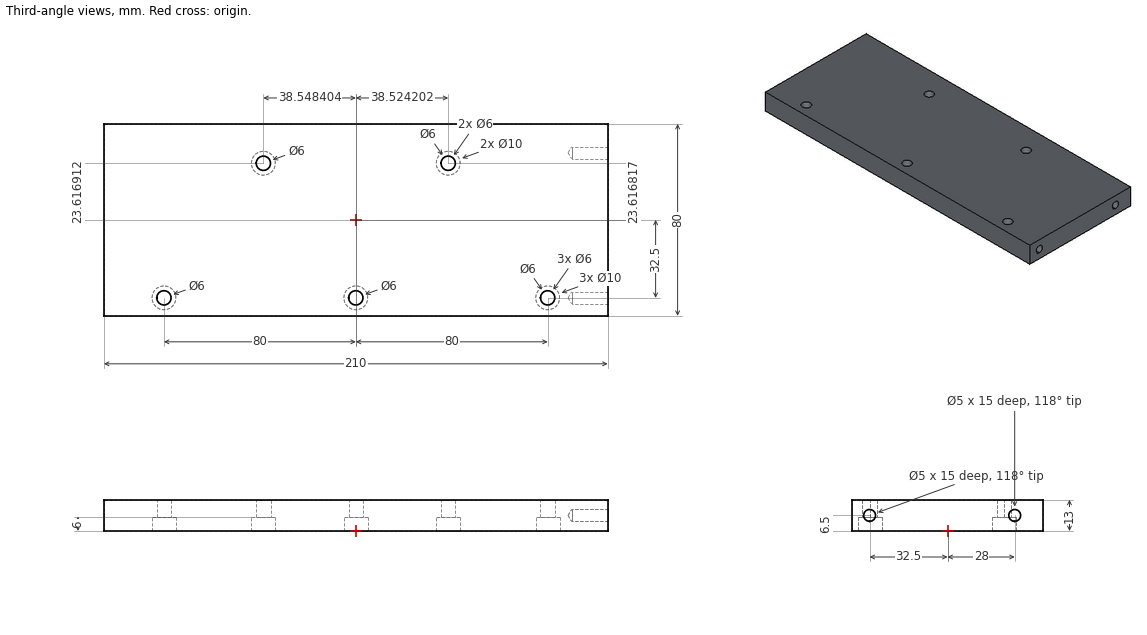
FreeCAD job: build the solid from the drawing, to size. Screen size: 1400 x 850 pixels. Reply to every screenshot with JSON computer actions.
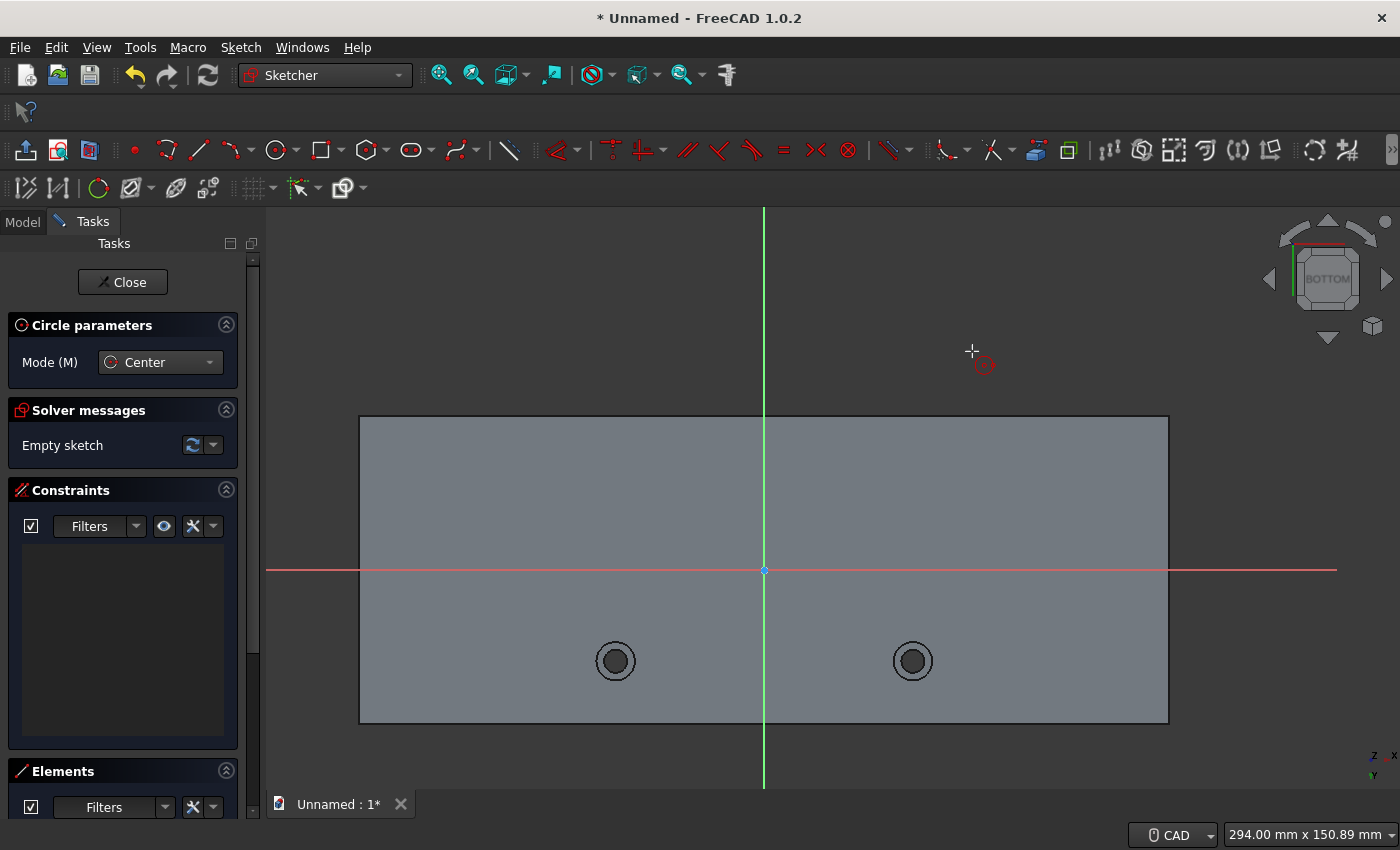
{"action": "left_click", "coordinate": [1073, 445]}
{"action": "left_click", "coordinate": [1087, 431]}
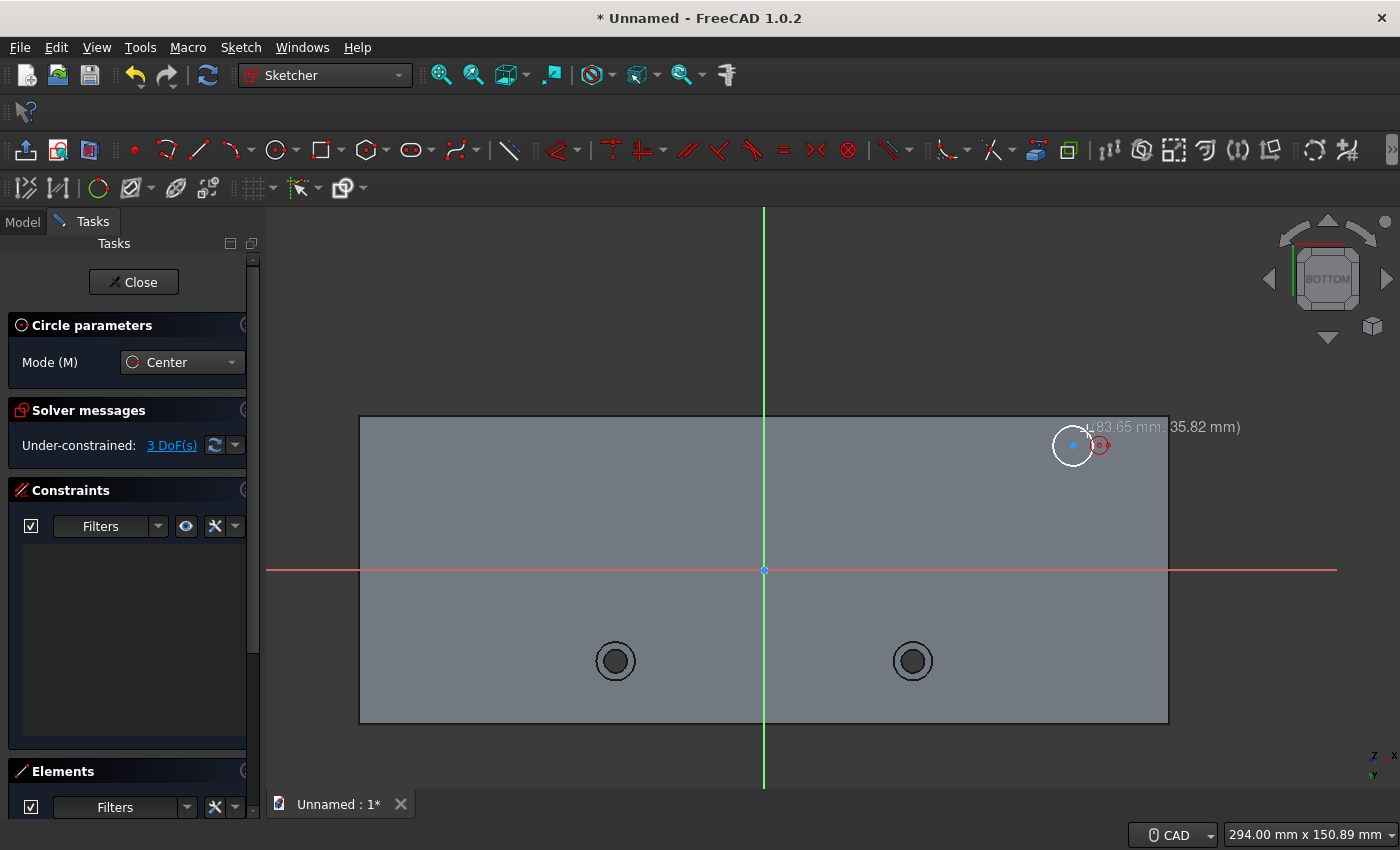
{"action": "left_click", "coordinate": [456, 445]}
{"action": "left_click", "coordinate": [469, 431]}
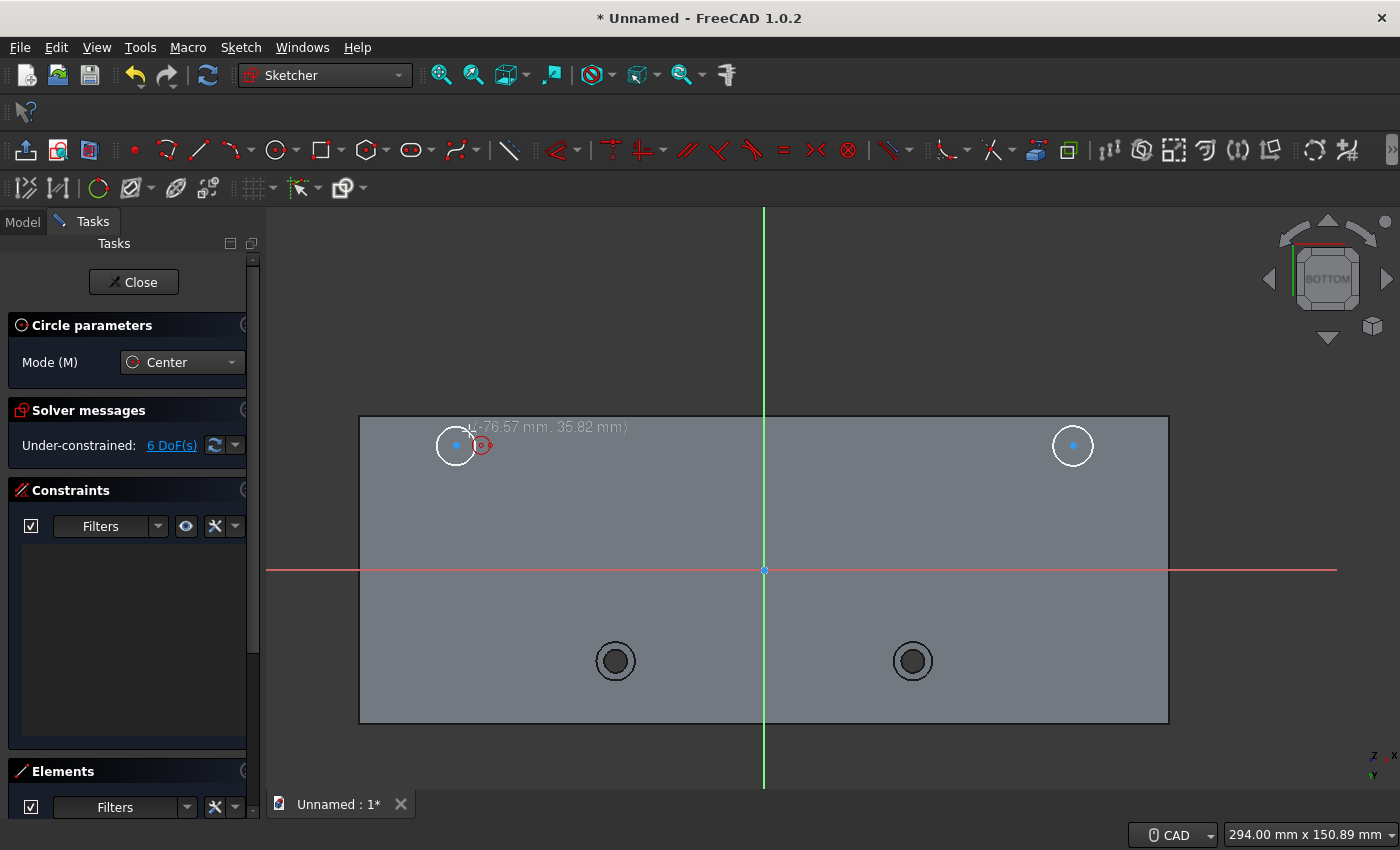
{"action": "left_click", "coordinate": [764, 445]}
{"action": "left_click", "coordinate": [782, 438]}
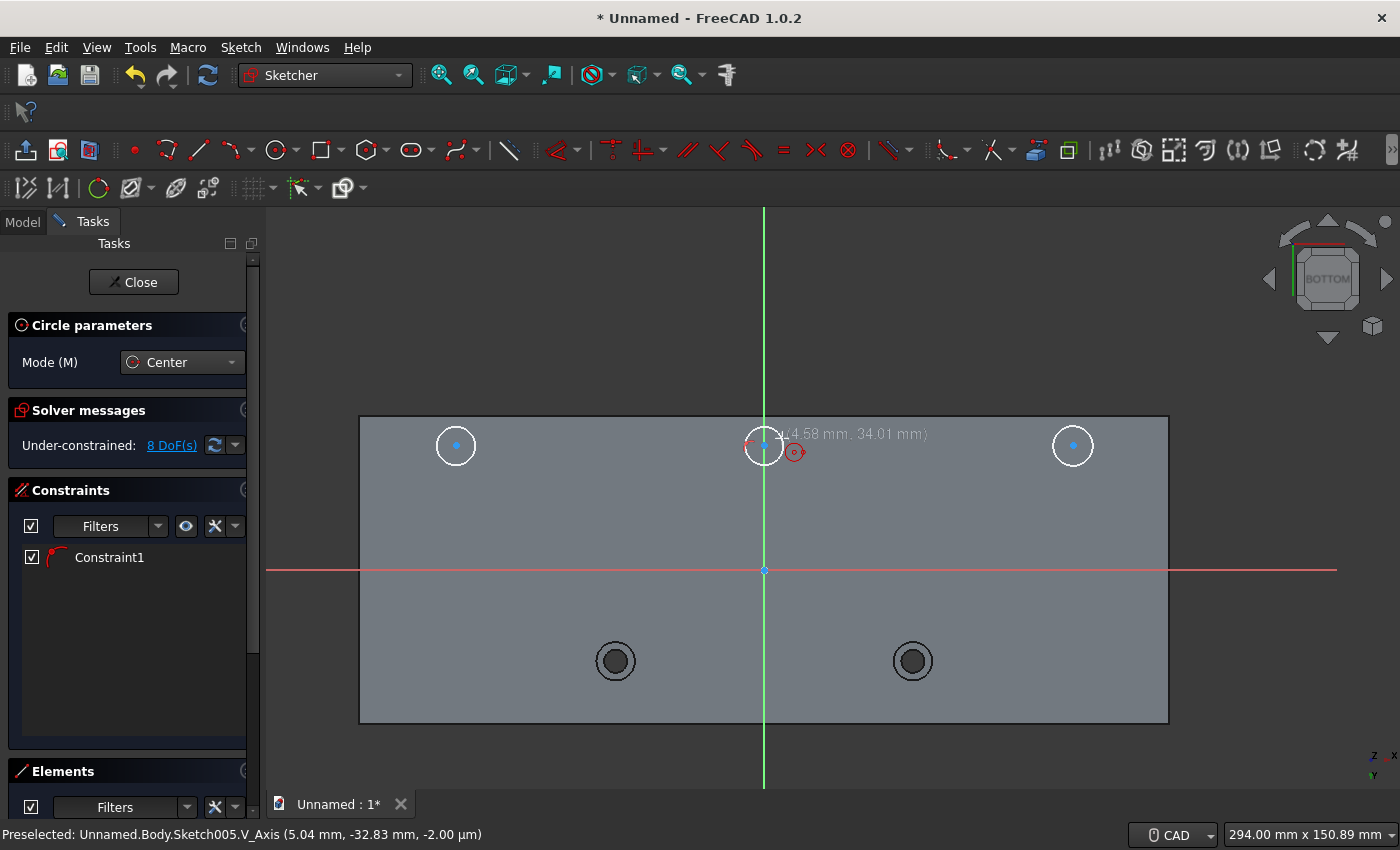
{"action": "scroll", "coordinate": [1073, 445], "scroll_direction": "up", "scroll_amount": 4}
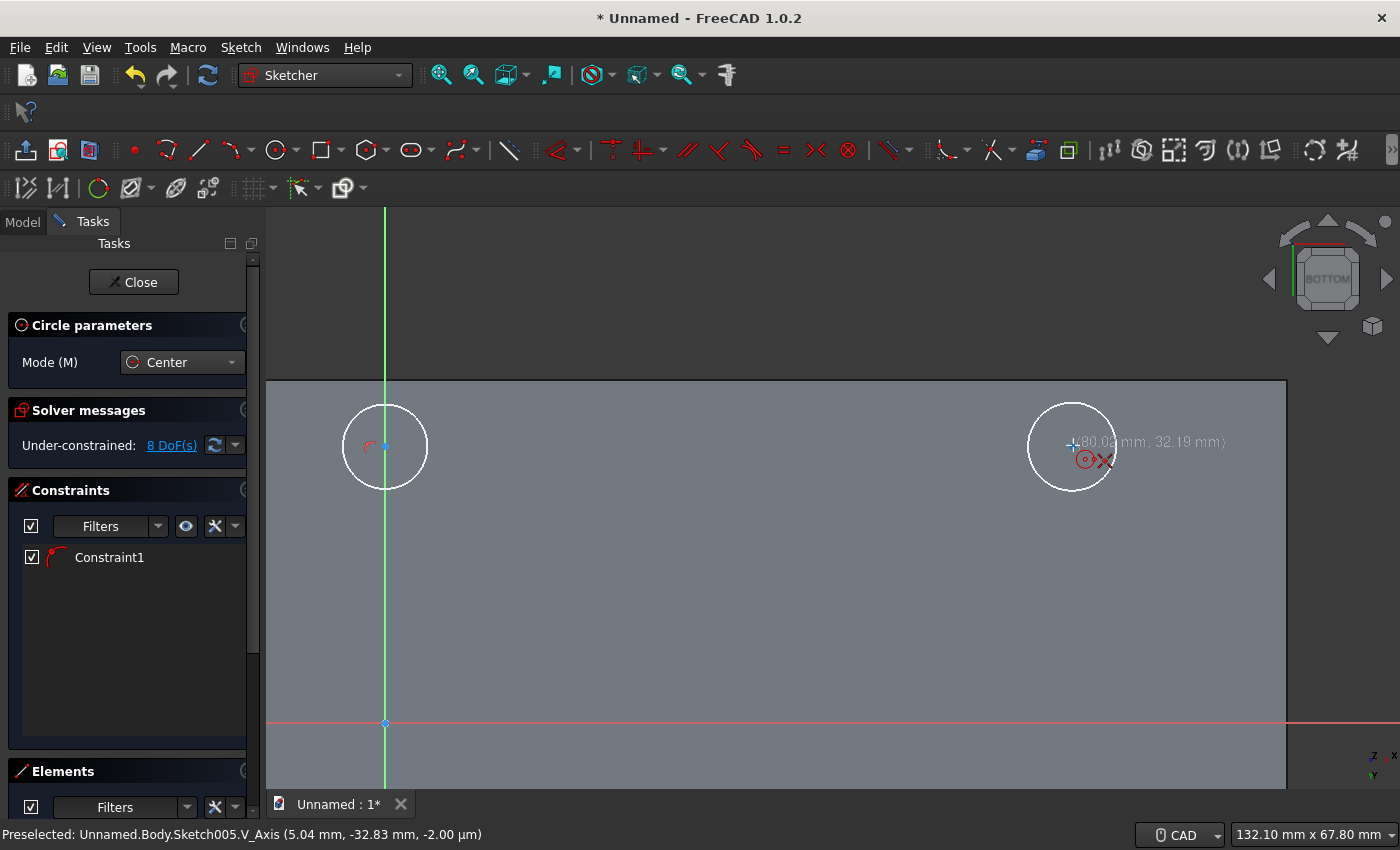
{"action": "left_click", "coordinate": [1072, 447]}
{"action": "left_click", "coordinate": [1090, 426]}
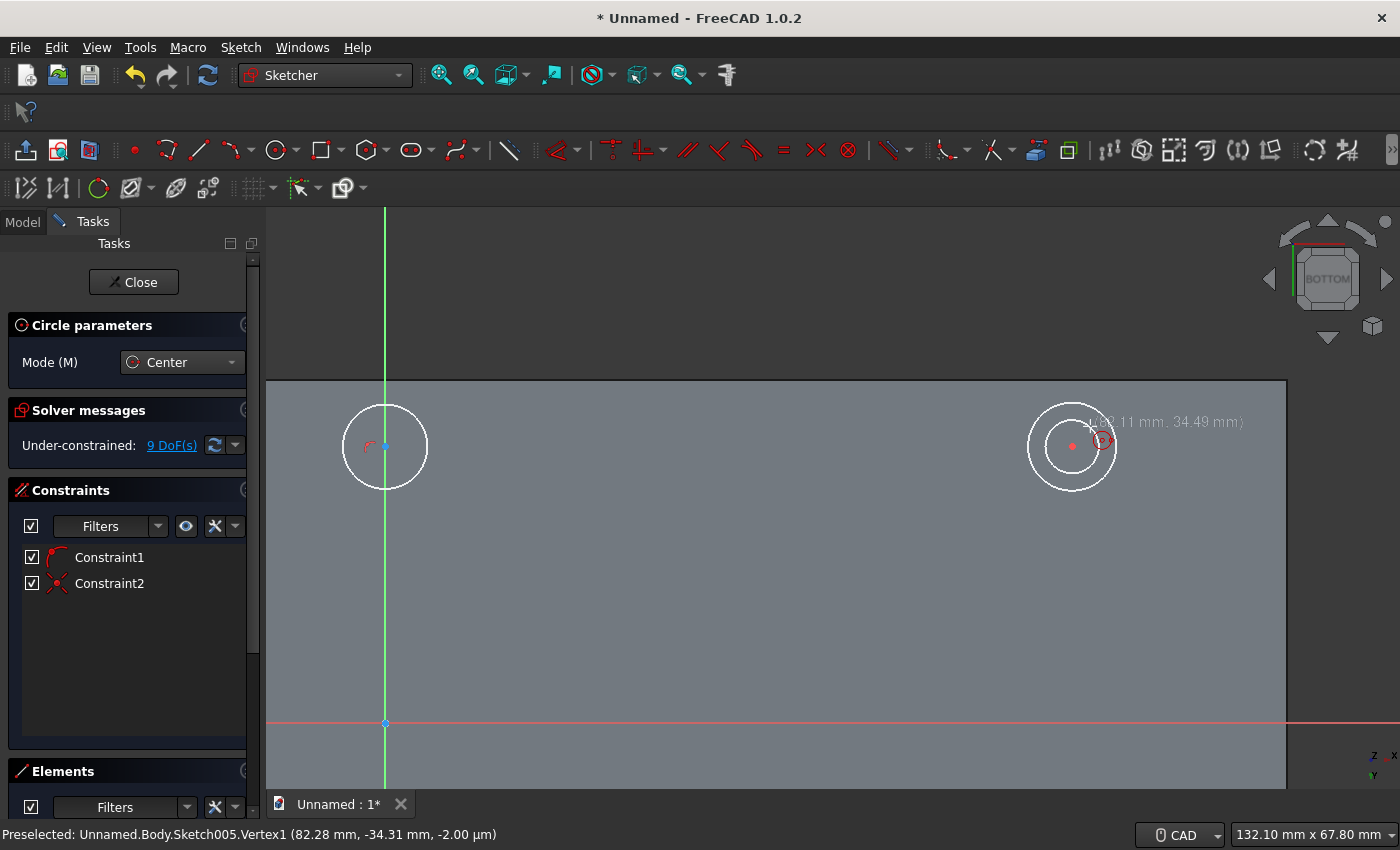
{"action": "scroll", "coordinate": [1074, 446], "scroll_direction": "down", "scroll_amount": 4}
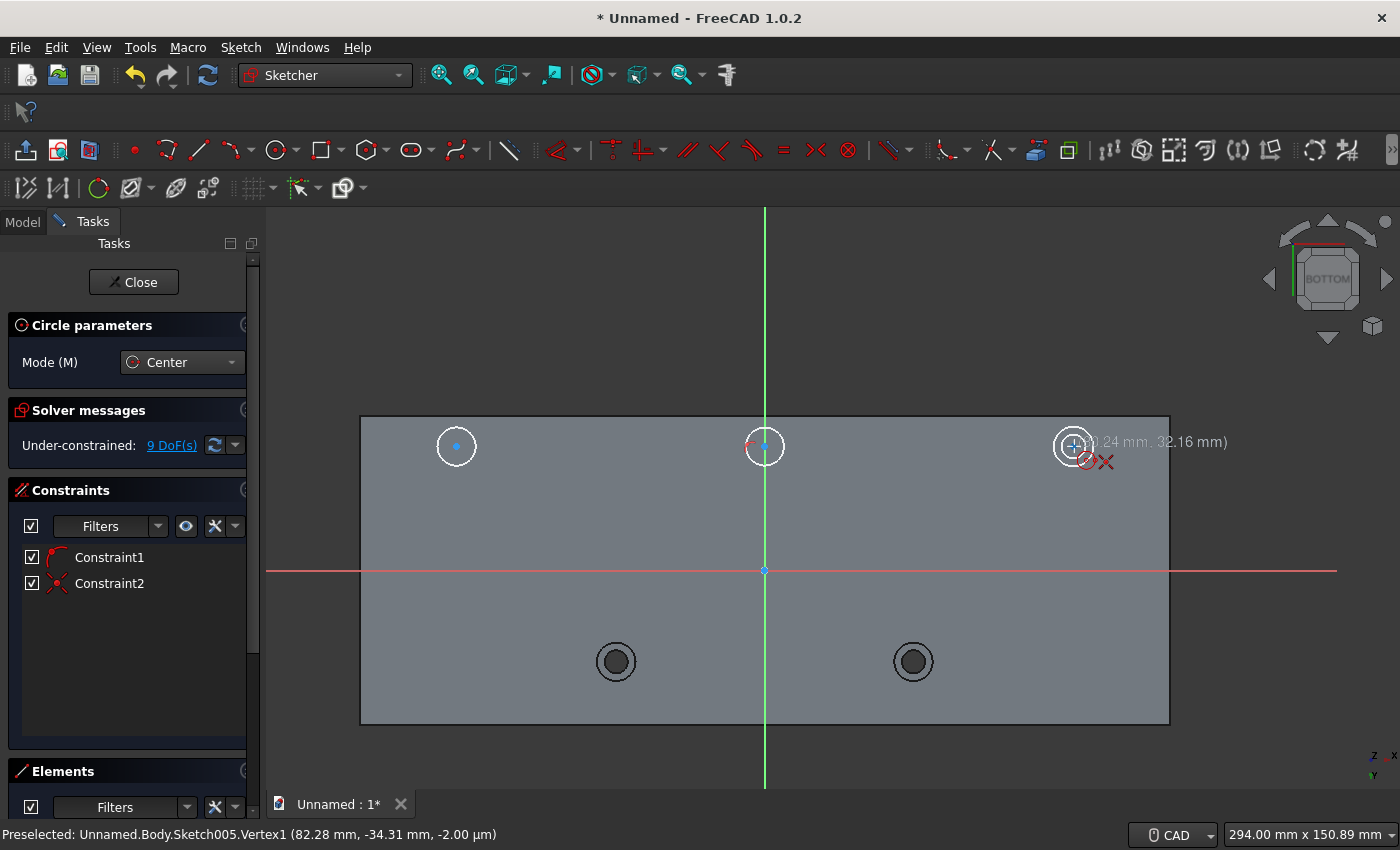
{"action": "scroll", "coordinate": [456, 445], "scroll_direction": "up", "scroll_amount": 4}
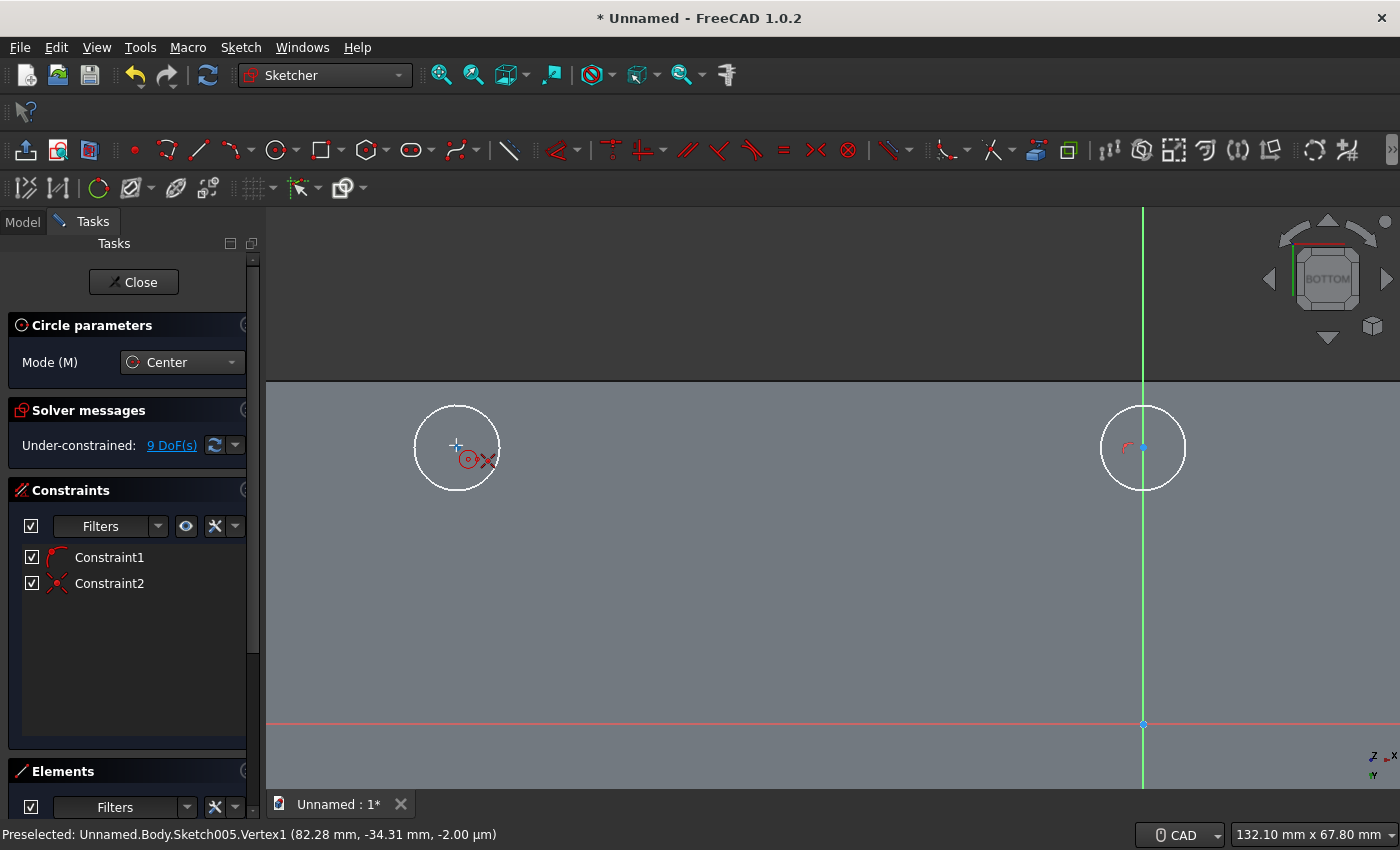
{"action": "left_click", "coordinate": [457, 448]}
{"action": "left_click", "coordinate": [475, 427]}